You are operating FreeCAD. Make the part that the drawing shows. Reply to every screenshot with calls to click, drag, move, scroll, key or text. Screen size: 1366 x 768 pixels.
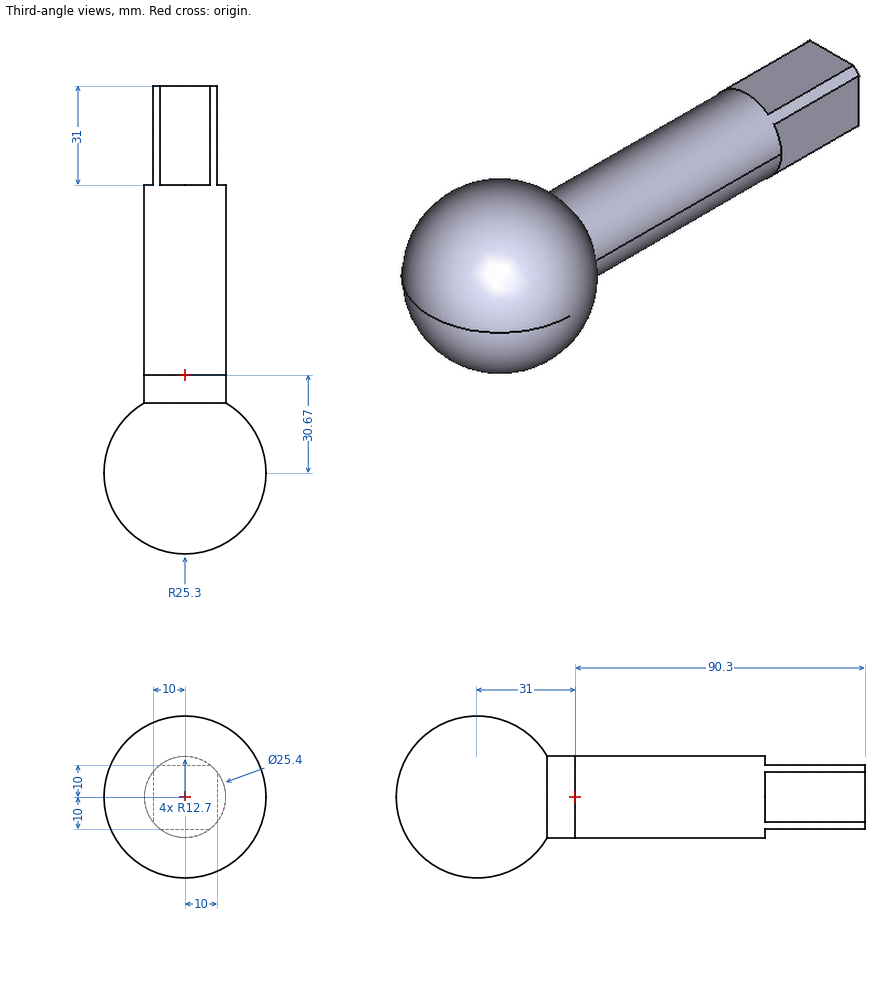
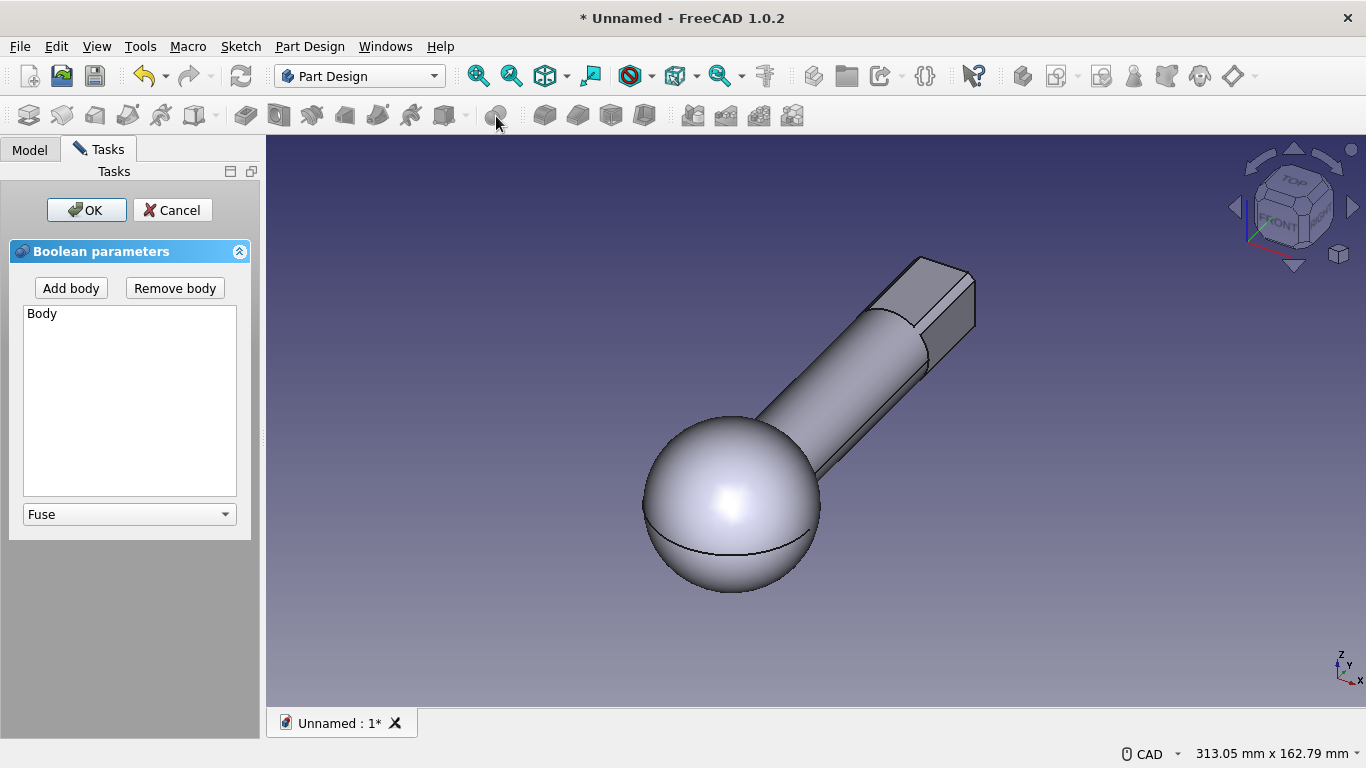
click(87, 210)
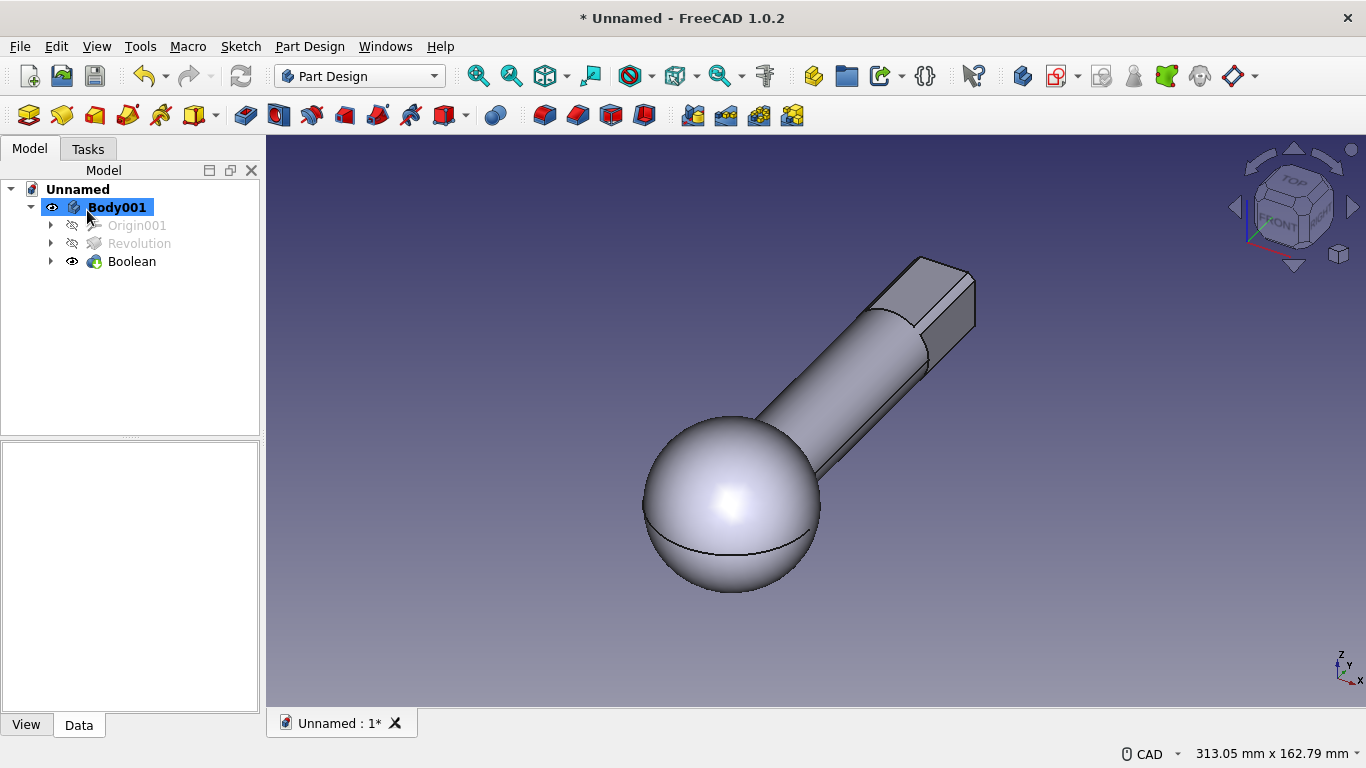
key(0)